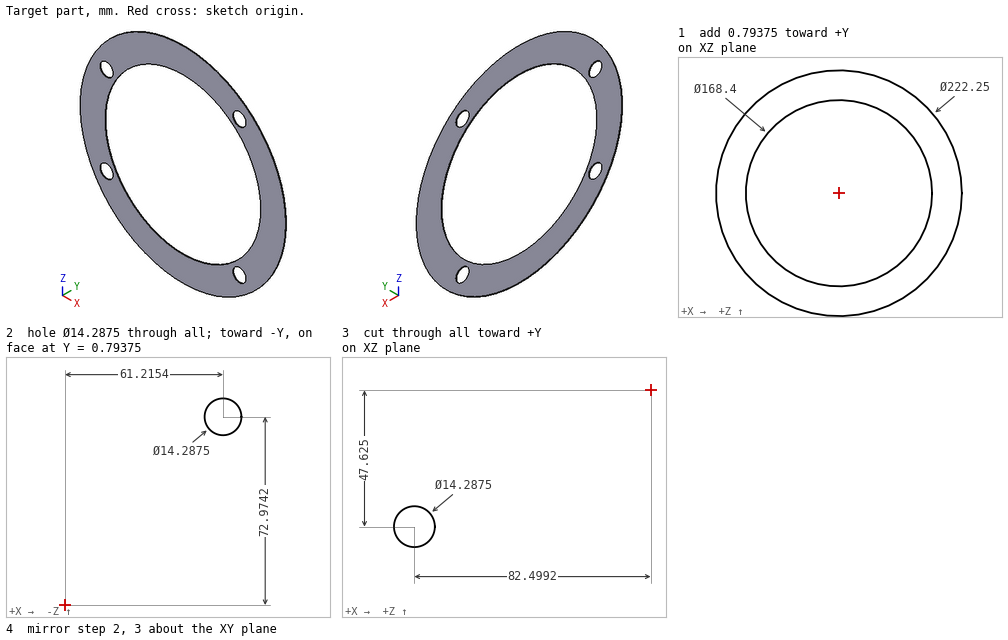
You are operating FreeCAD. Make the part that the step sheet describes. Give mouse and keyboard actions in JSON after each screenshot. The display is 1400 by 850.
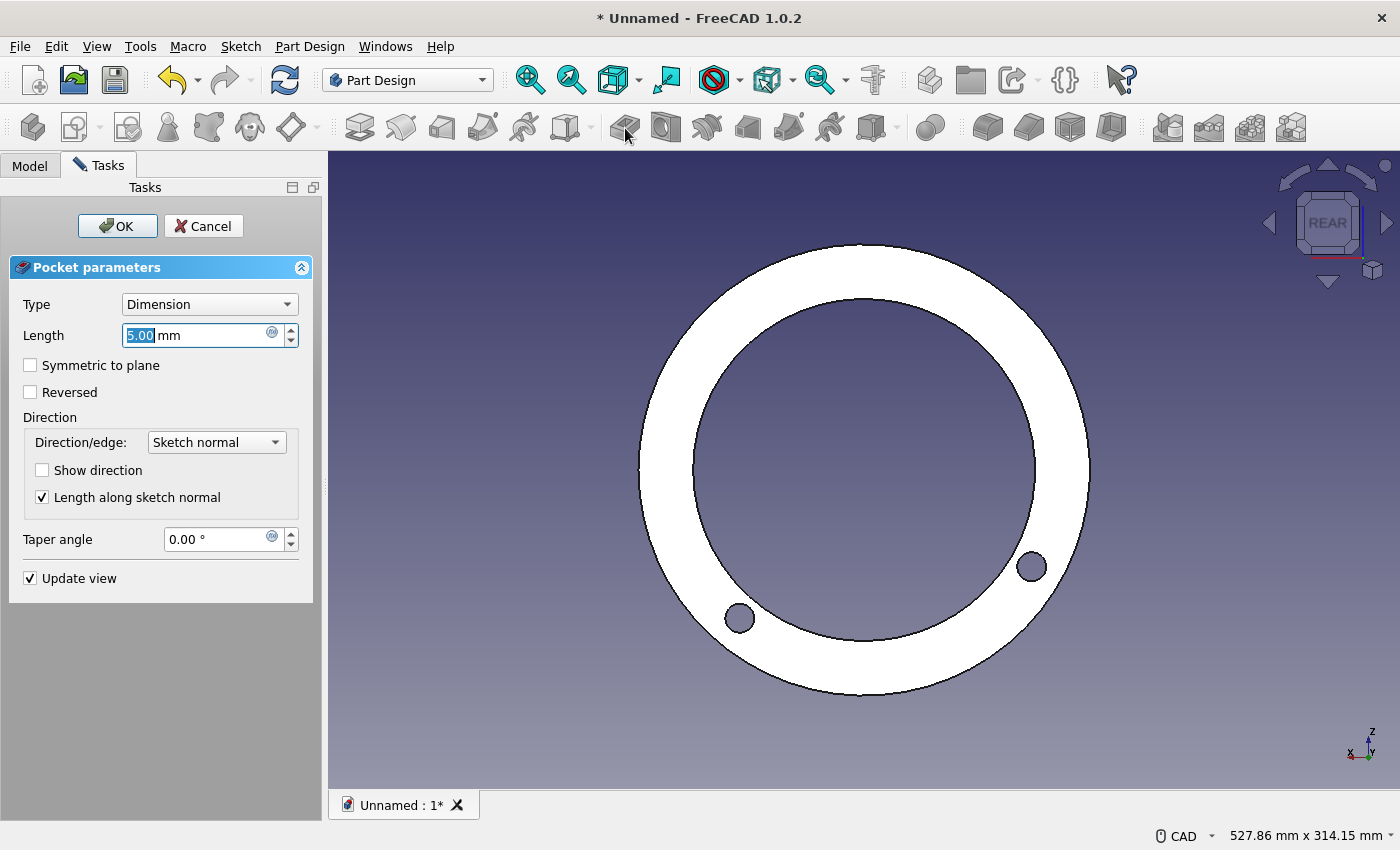
{"action": "left_click", "coordinate": [210, 304]}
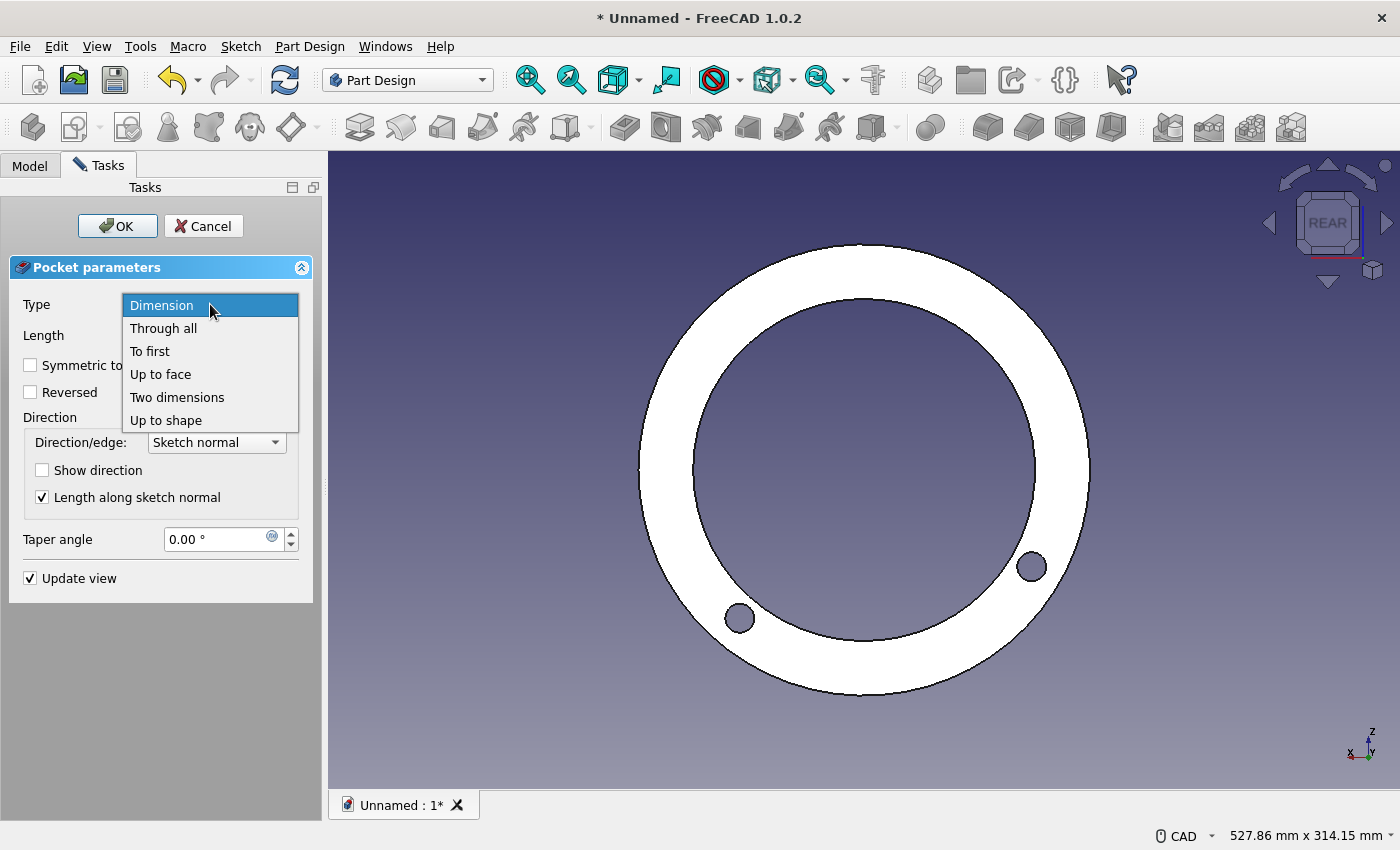
{"action": "left_click", "coordinate": [208, 328]}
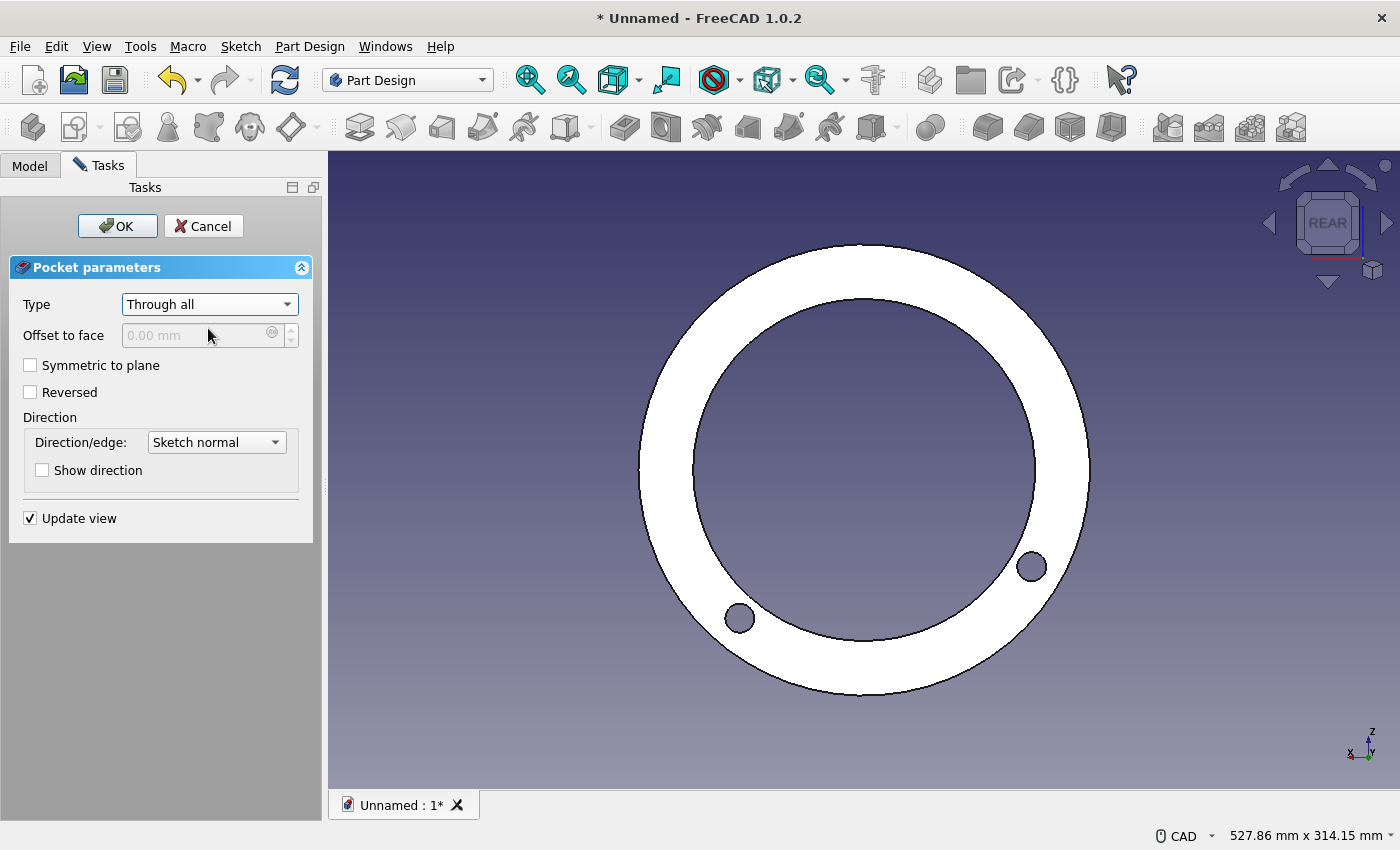
{"action": "left_click", "coordinate": [118, 226]}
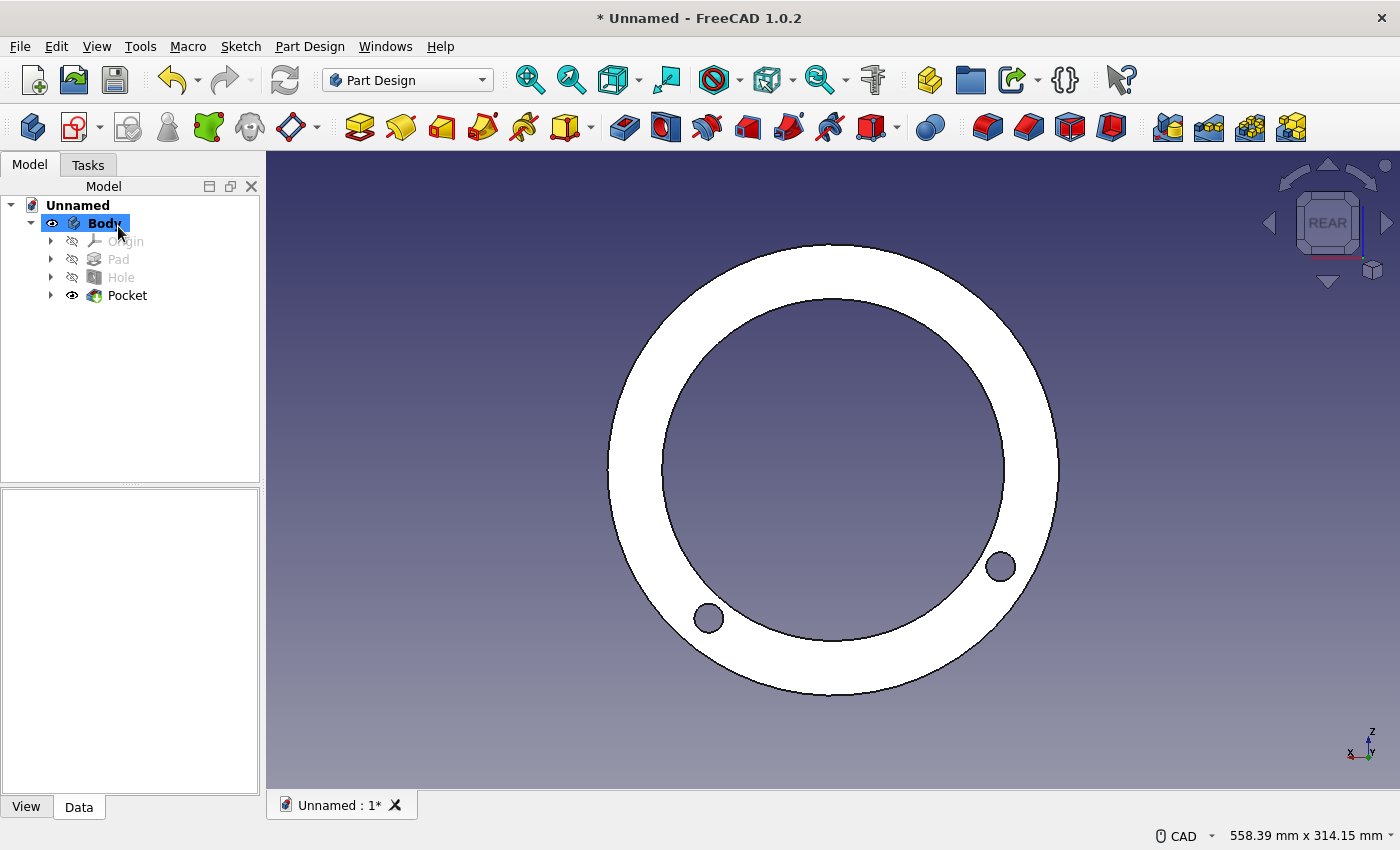
{"action": "left_click", "coordinate": [117, 277]}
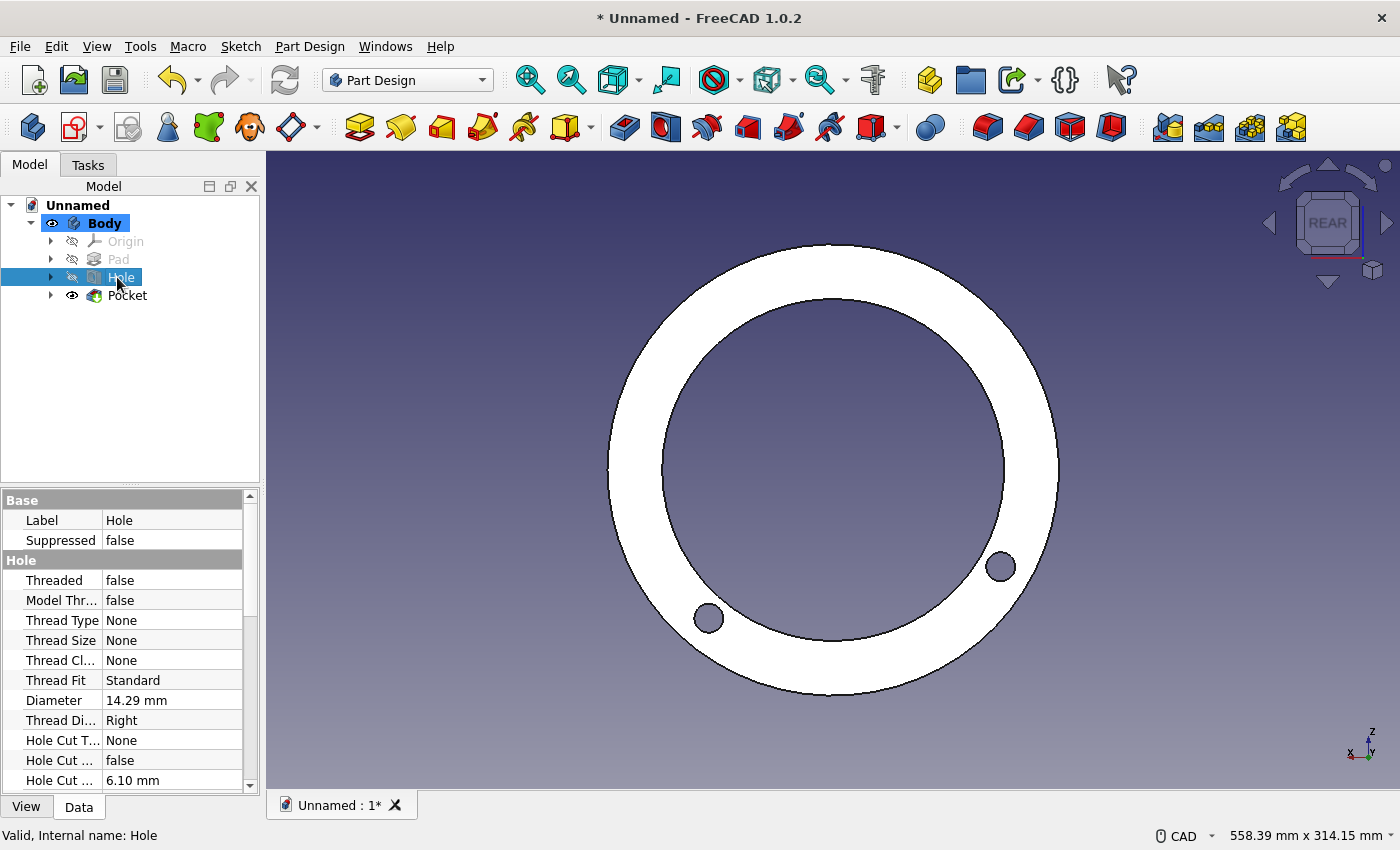
{"action": "left_click", "coordinate": [117, 295], "text": "ctrl"}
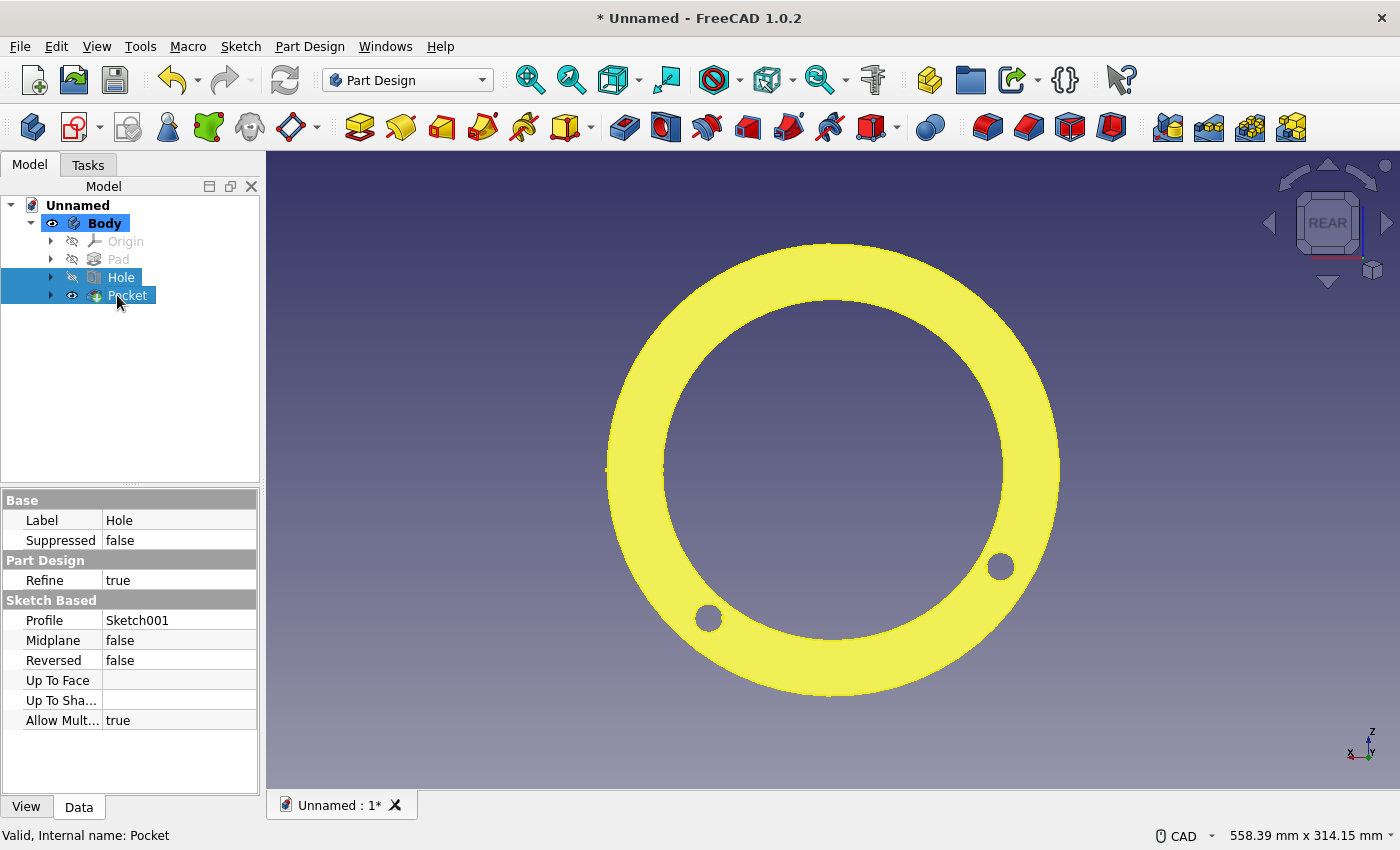
{"action": "left_click", "coordinate": [1168, 128]}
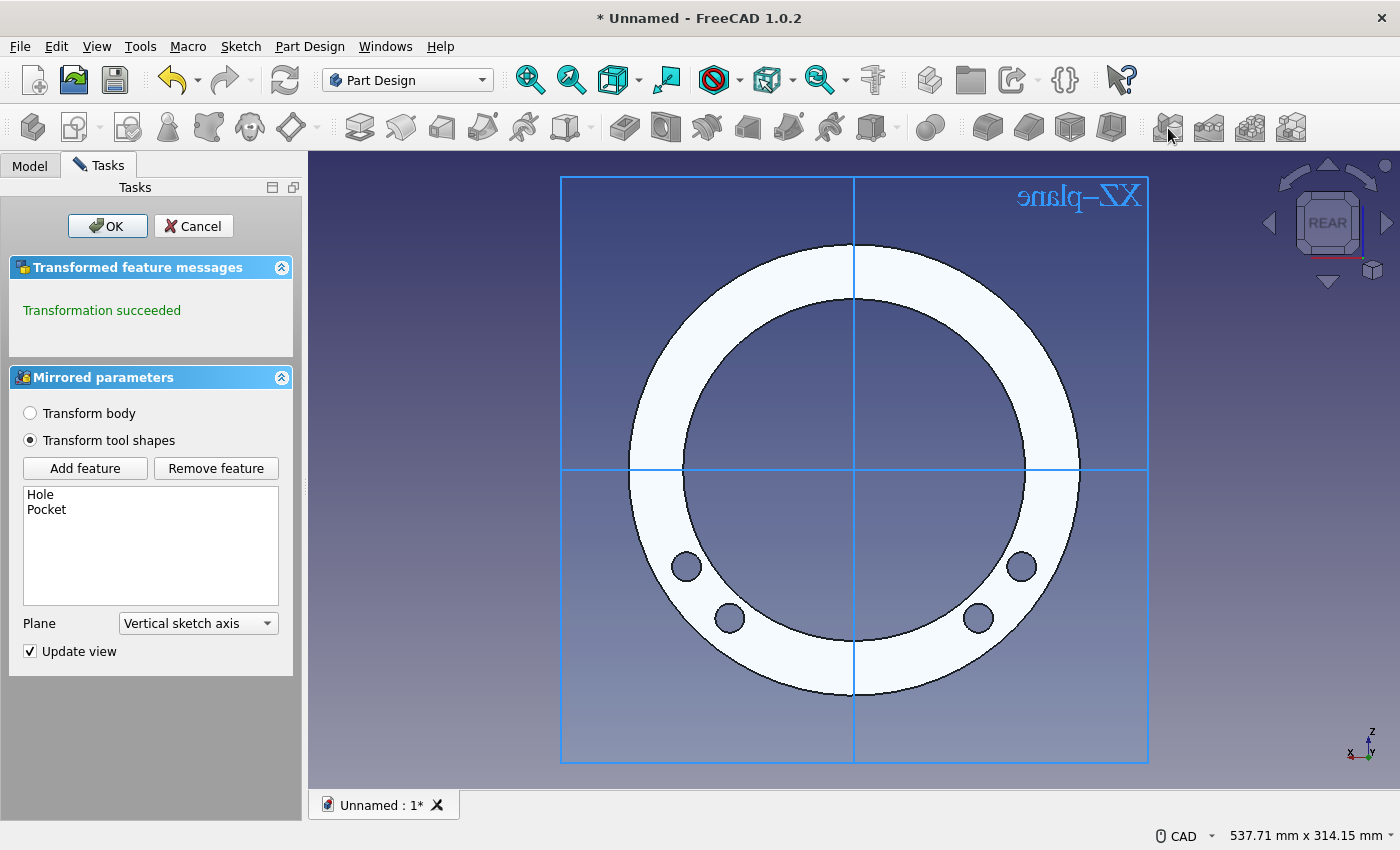
{"action": "left_click", "coordinate": [199, 624]}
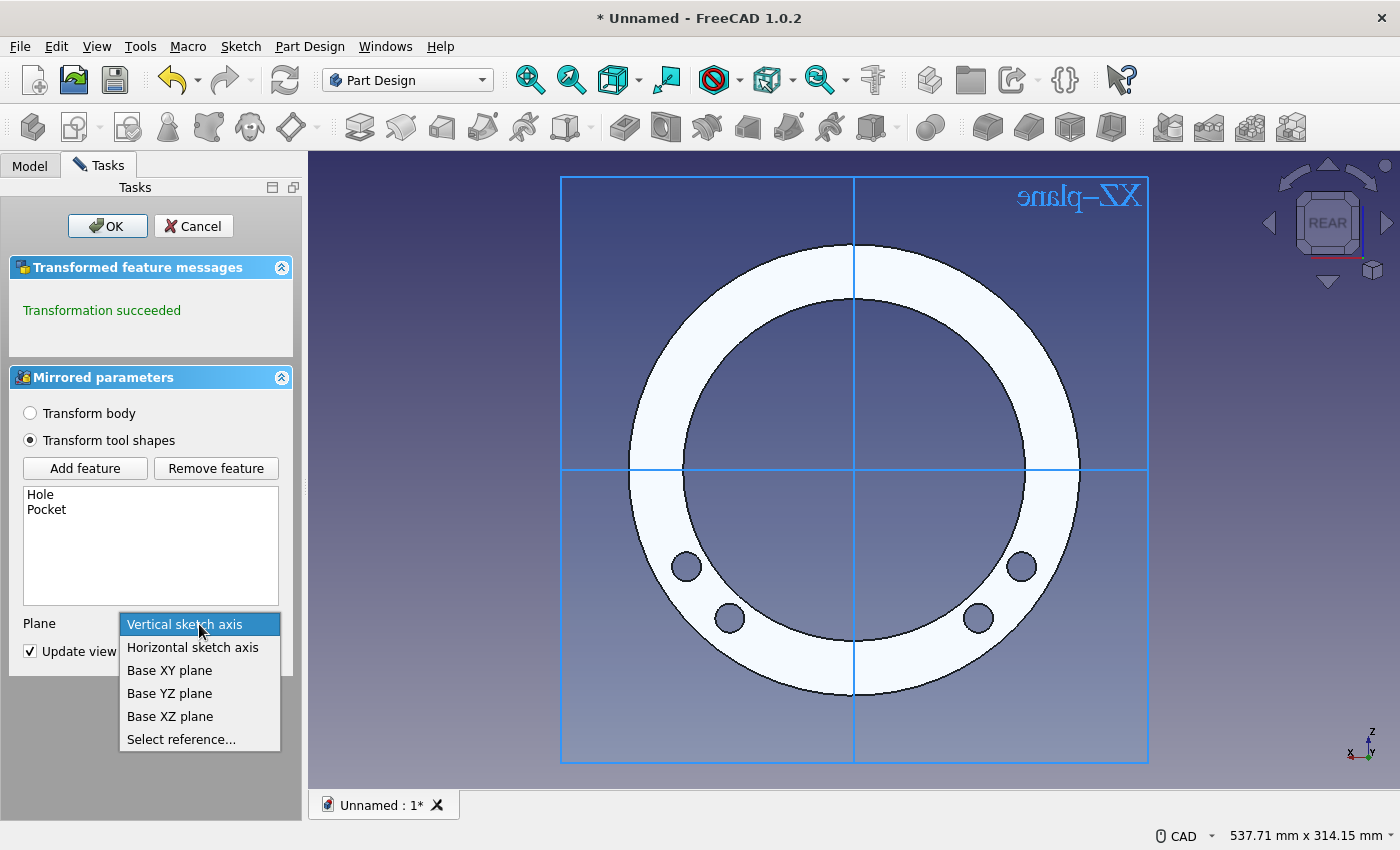
{"action": "left_click", "coordinate": [198, 670]}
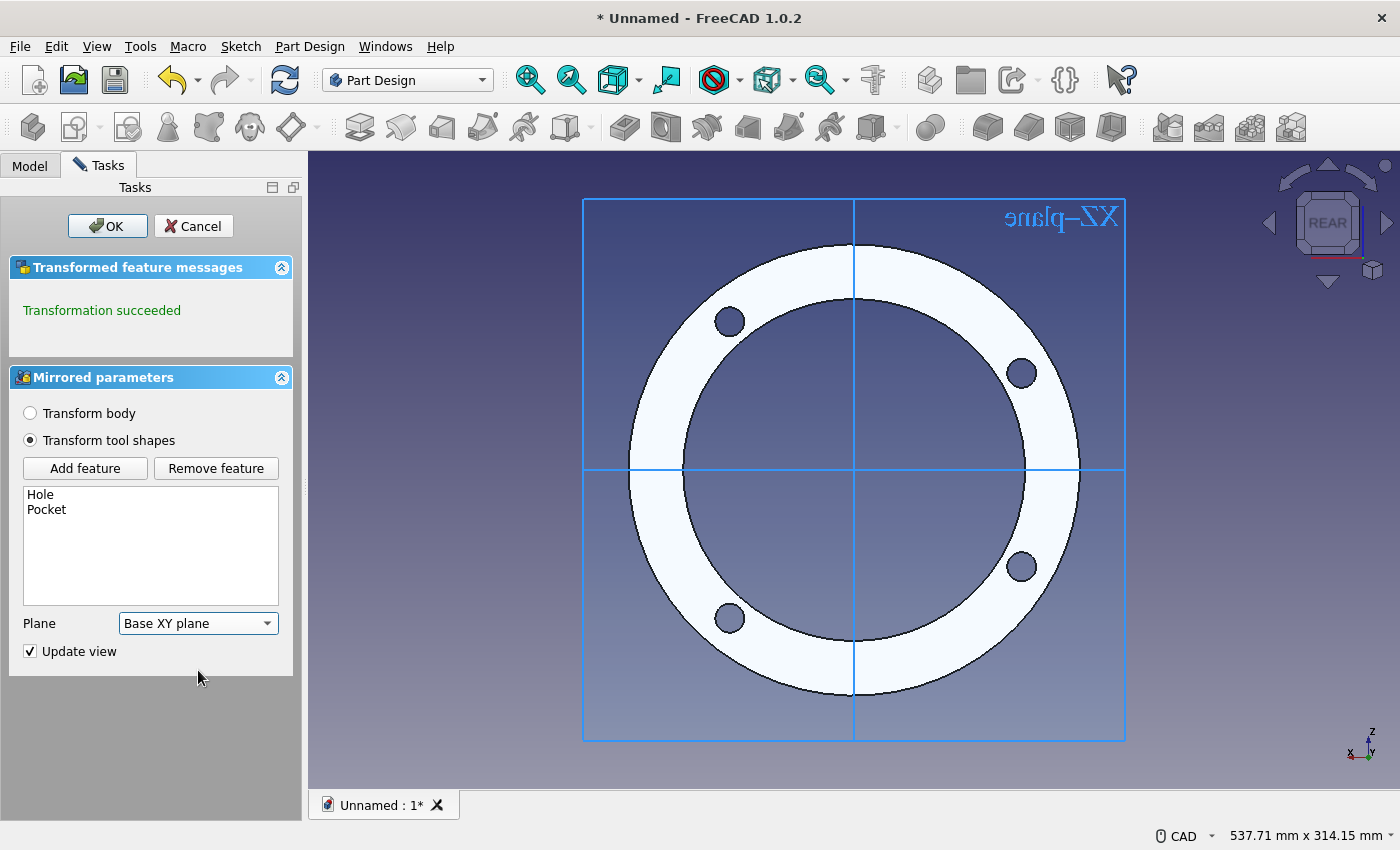
{"action": "left_click", "coordinate": [108, 226]}